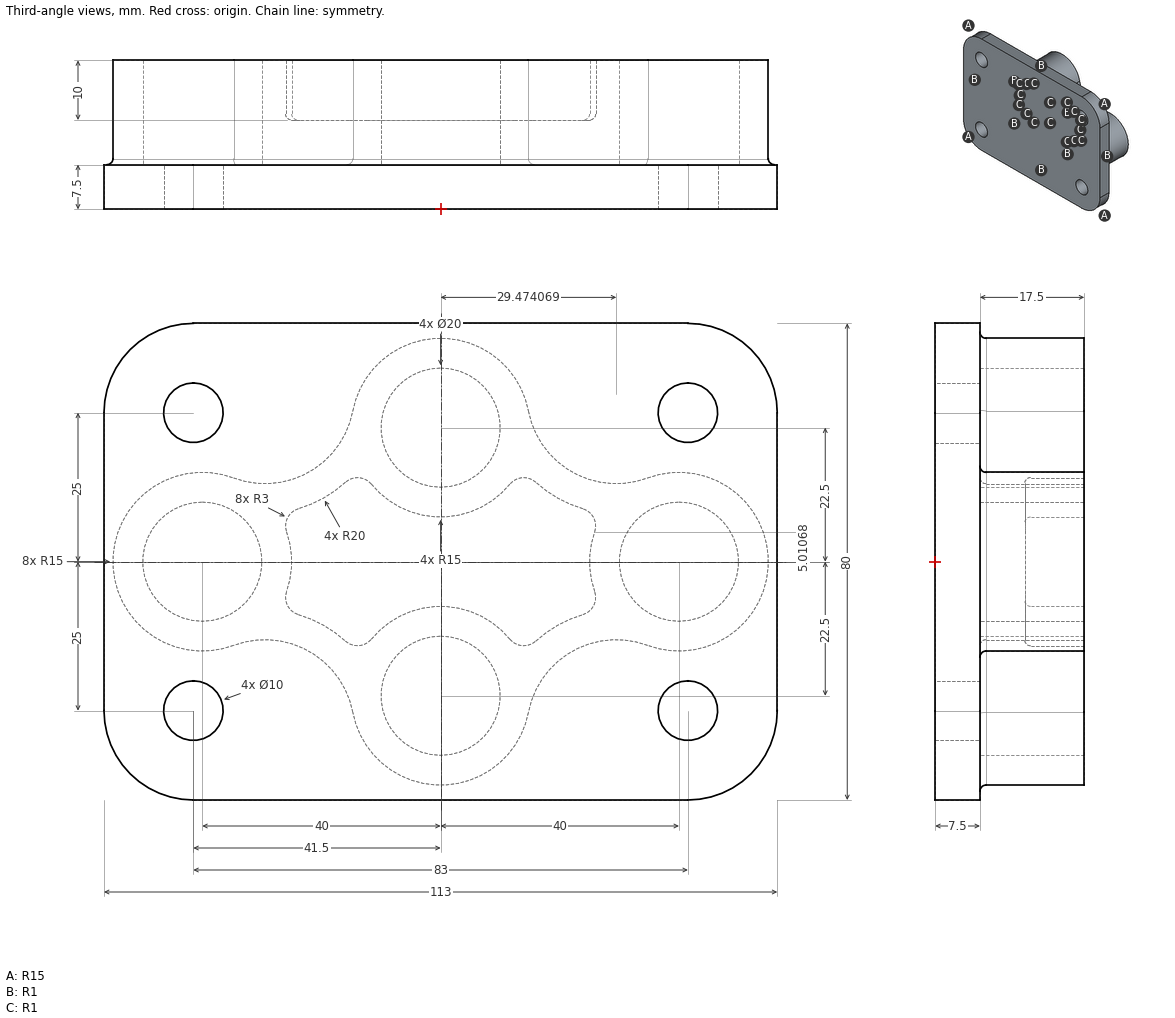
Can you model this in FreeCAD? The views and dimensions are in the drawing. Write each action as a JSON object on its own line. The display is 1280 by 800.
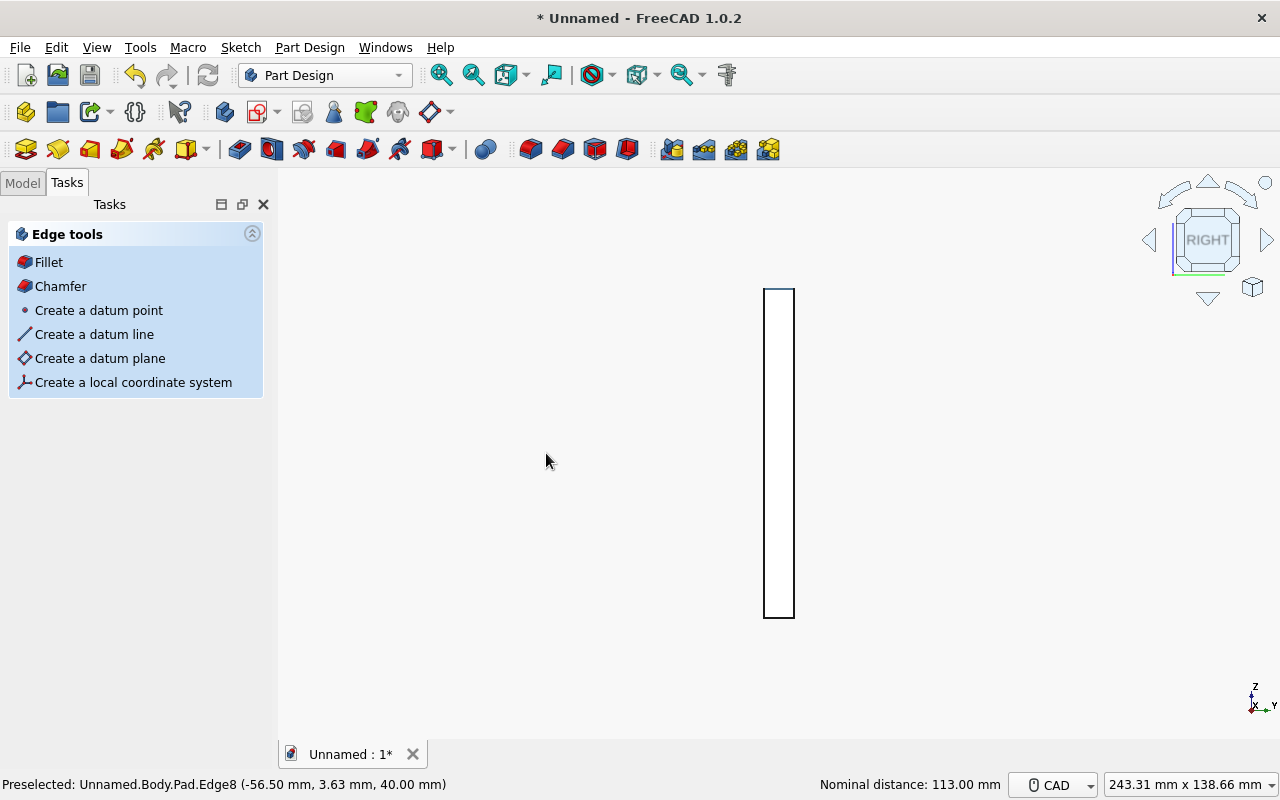
{"action": "left_click", "coordinate": [779, 617], "text": "ctrl"}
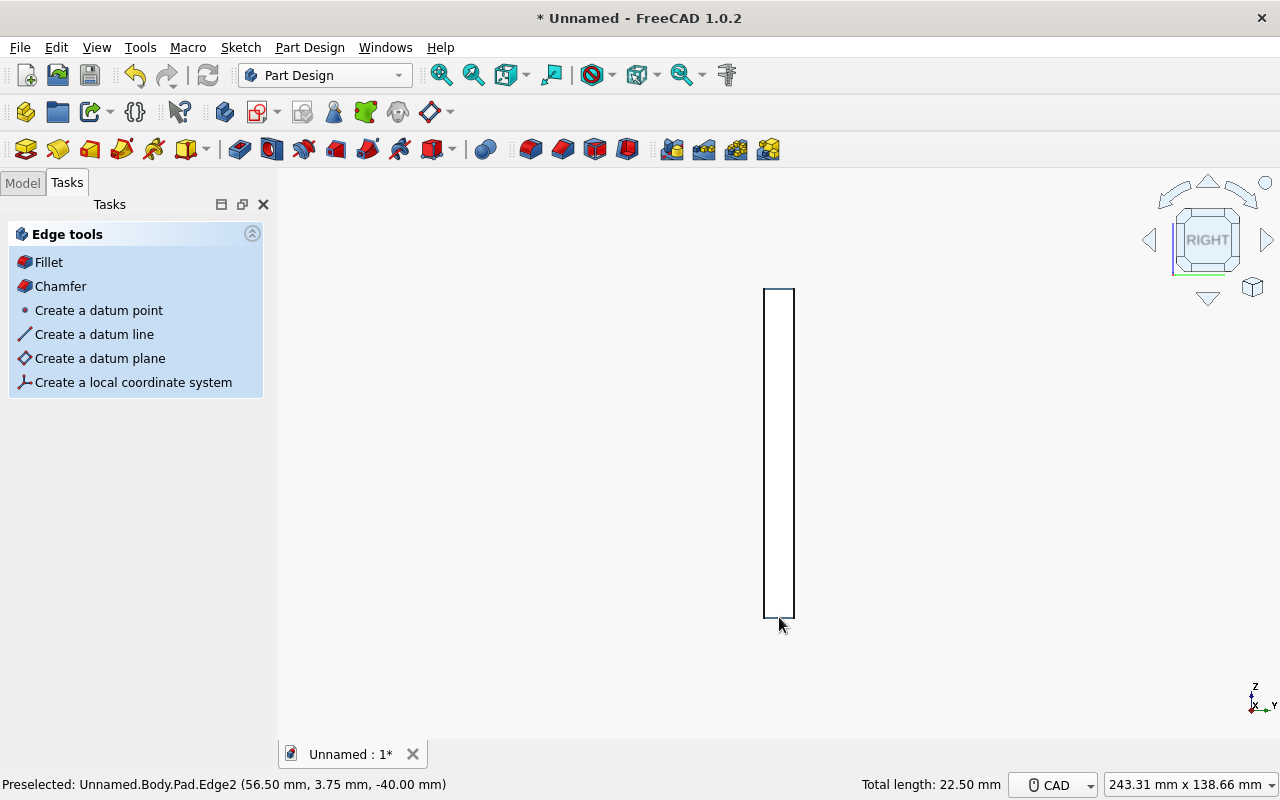
{"action": "key", "text": "5"}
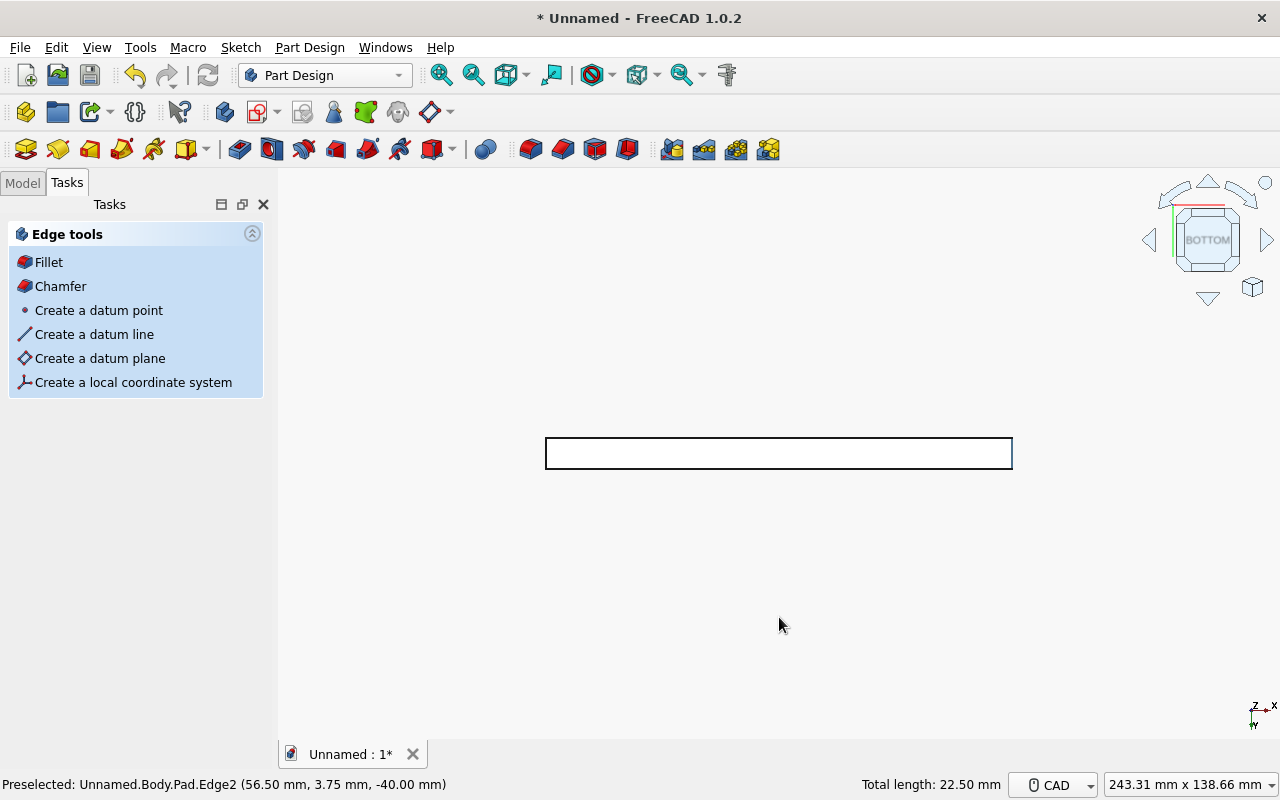
{"action": "left_click", "coordinate": [546, 453], "text": "ctrl"}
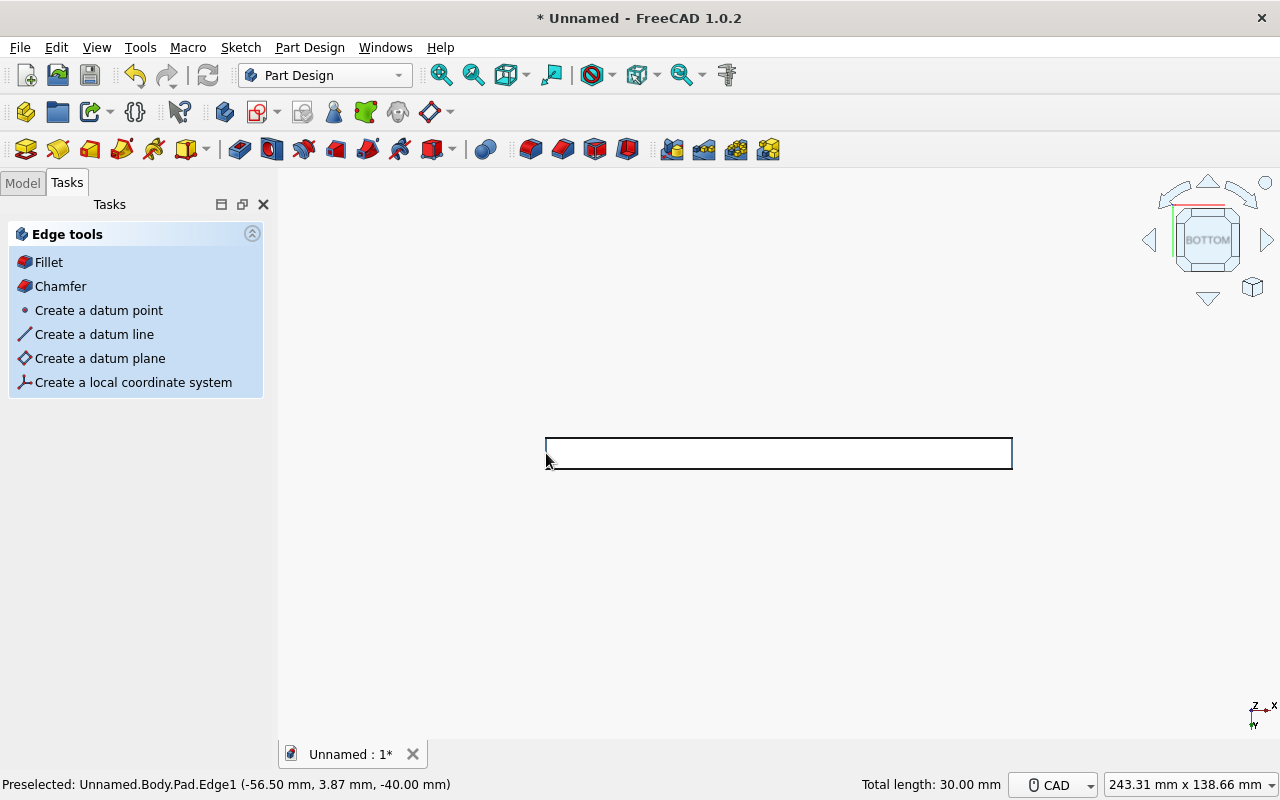
{"action": "left_click", "coordinate": [532, 150]}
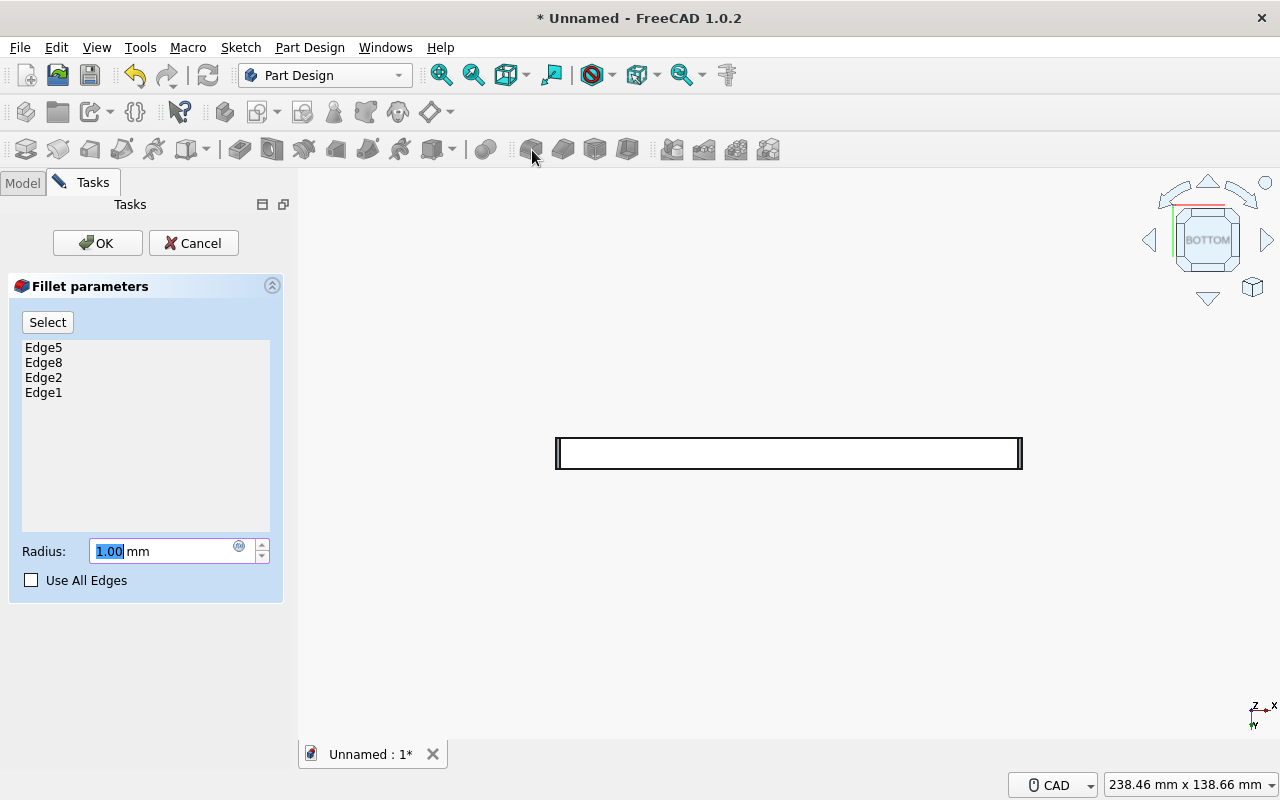
{"action": "type", "text": "15"}
{"action": "key", "text": "Tab"}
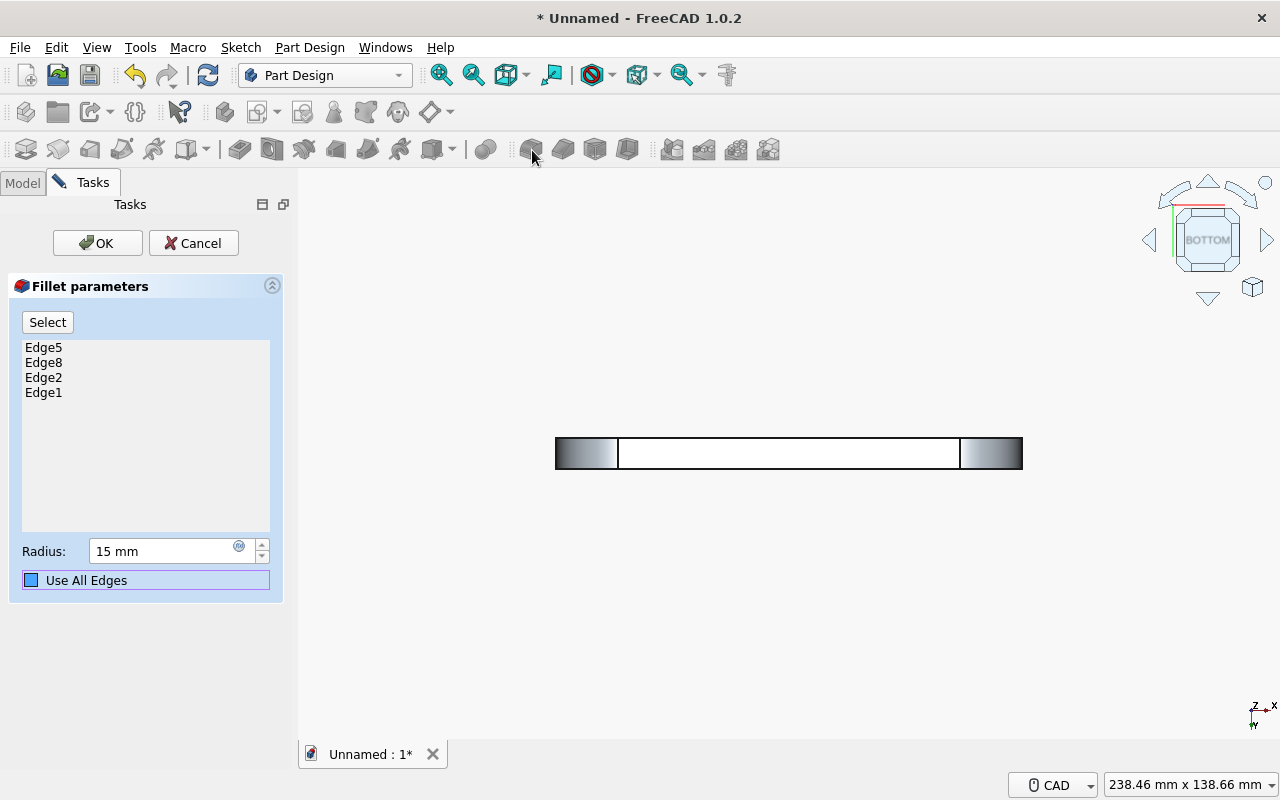
{"action": "left_click", "coordinate": [98, 243]}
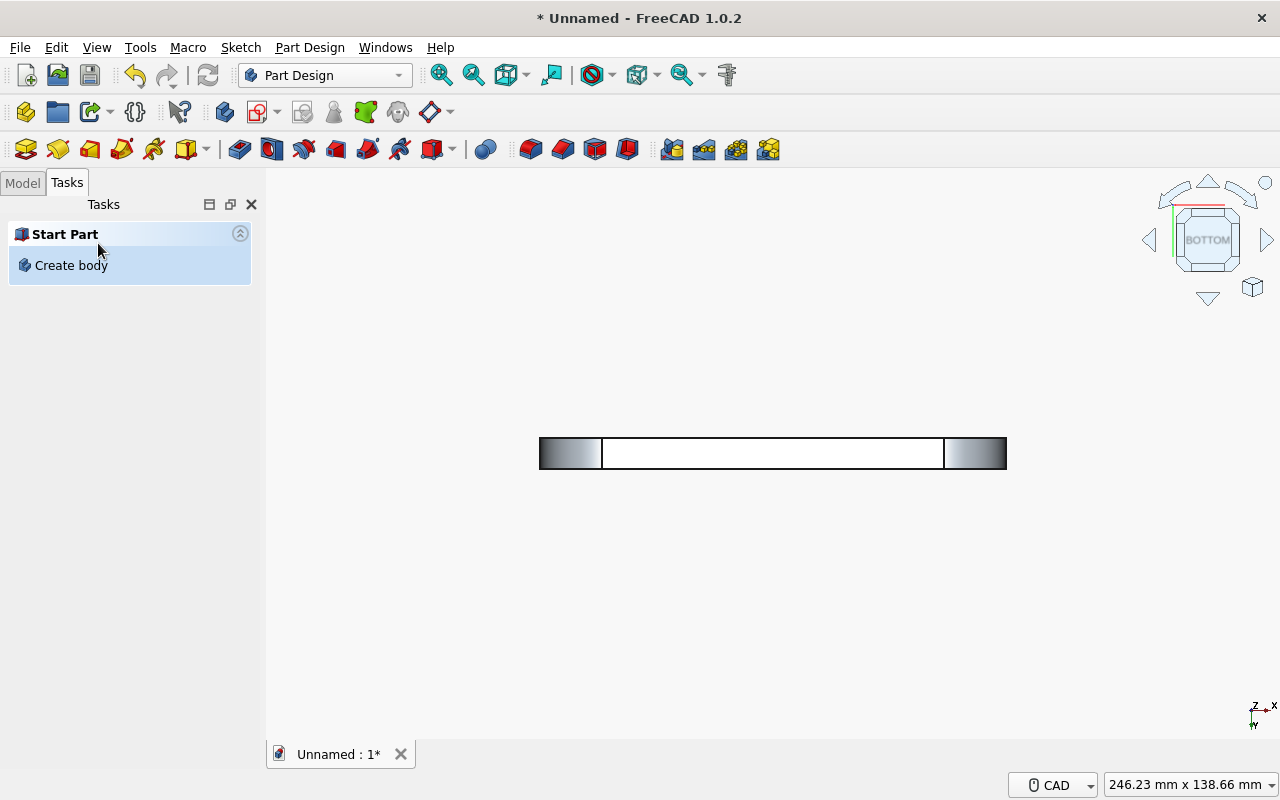
{"action": "key", "text": "4"}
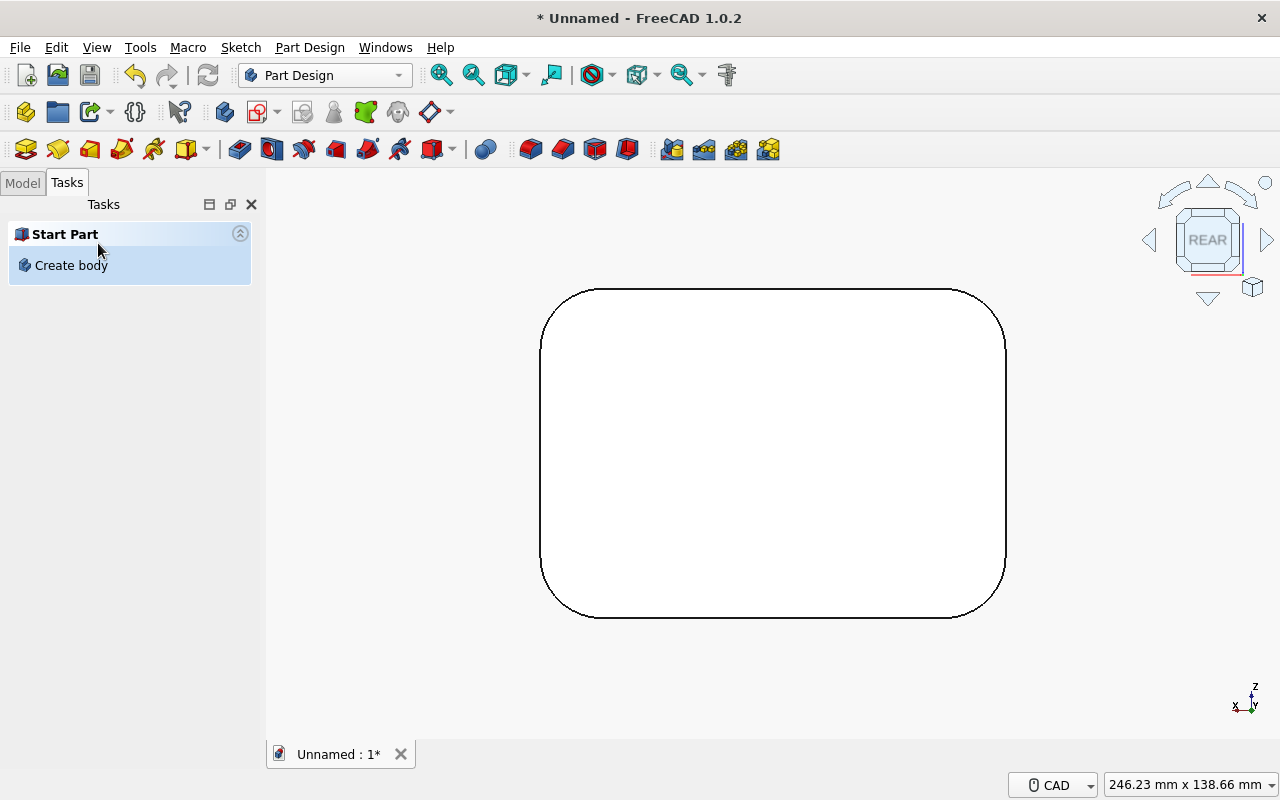
{"action": "left_click", "coordinate": [707, 452]}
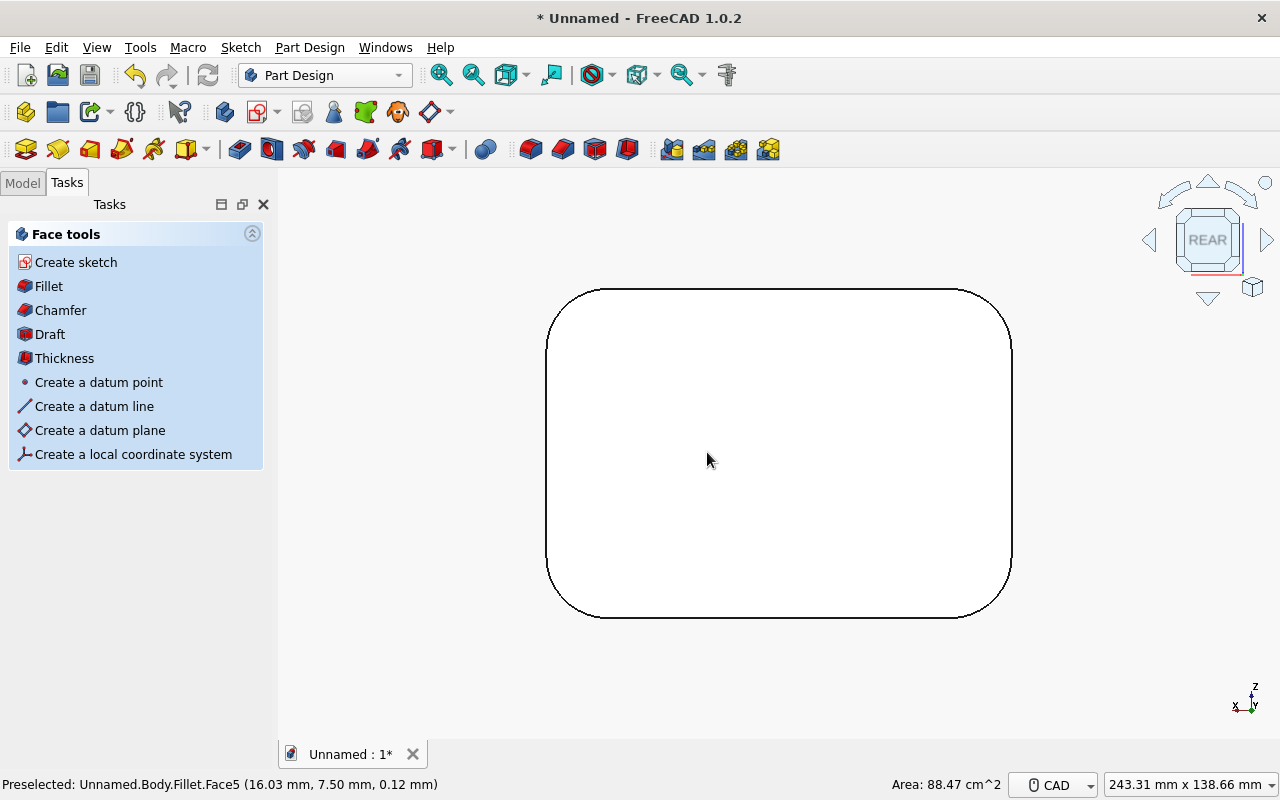
{"action": "left_click", "coordinate": [258, 112]}